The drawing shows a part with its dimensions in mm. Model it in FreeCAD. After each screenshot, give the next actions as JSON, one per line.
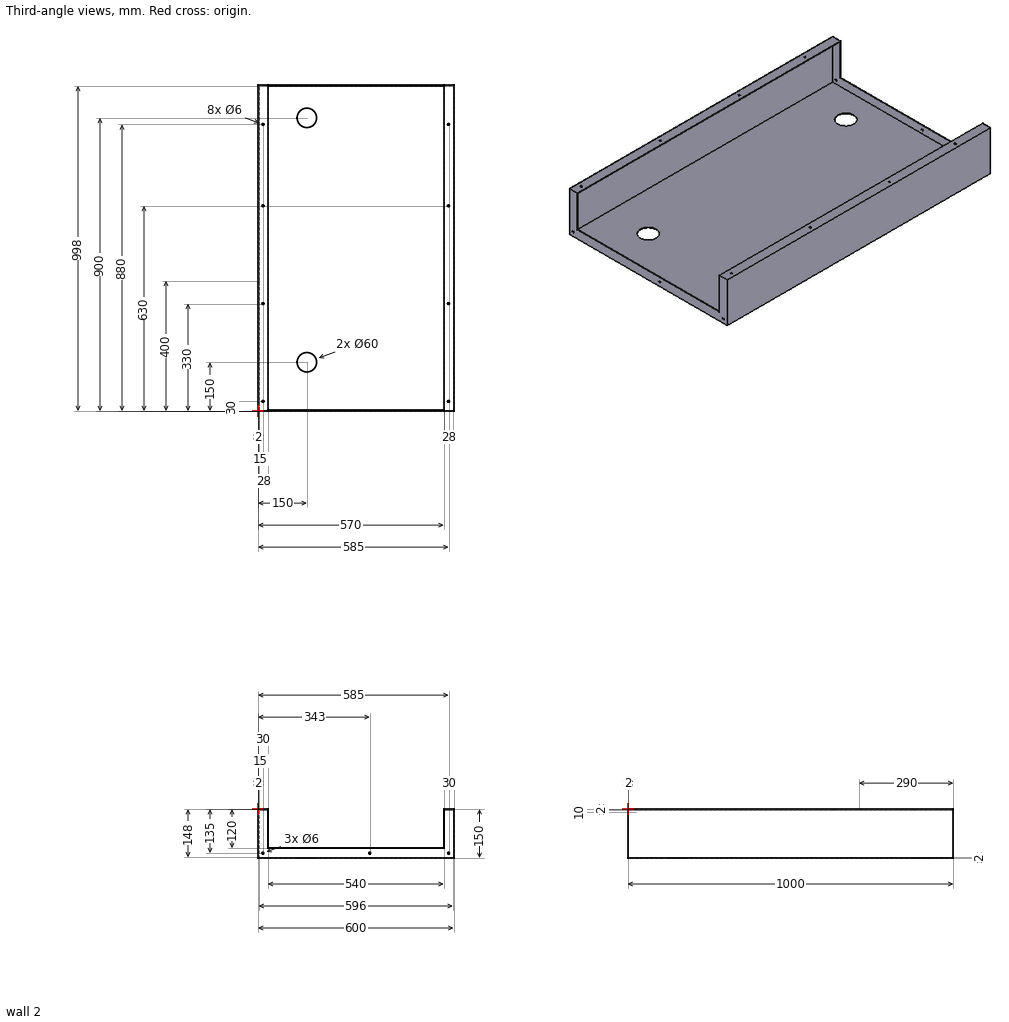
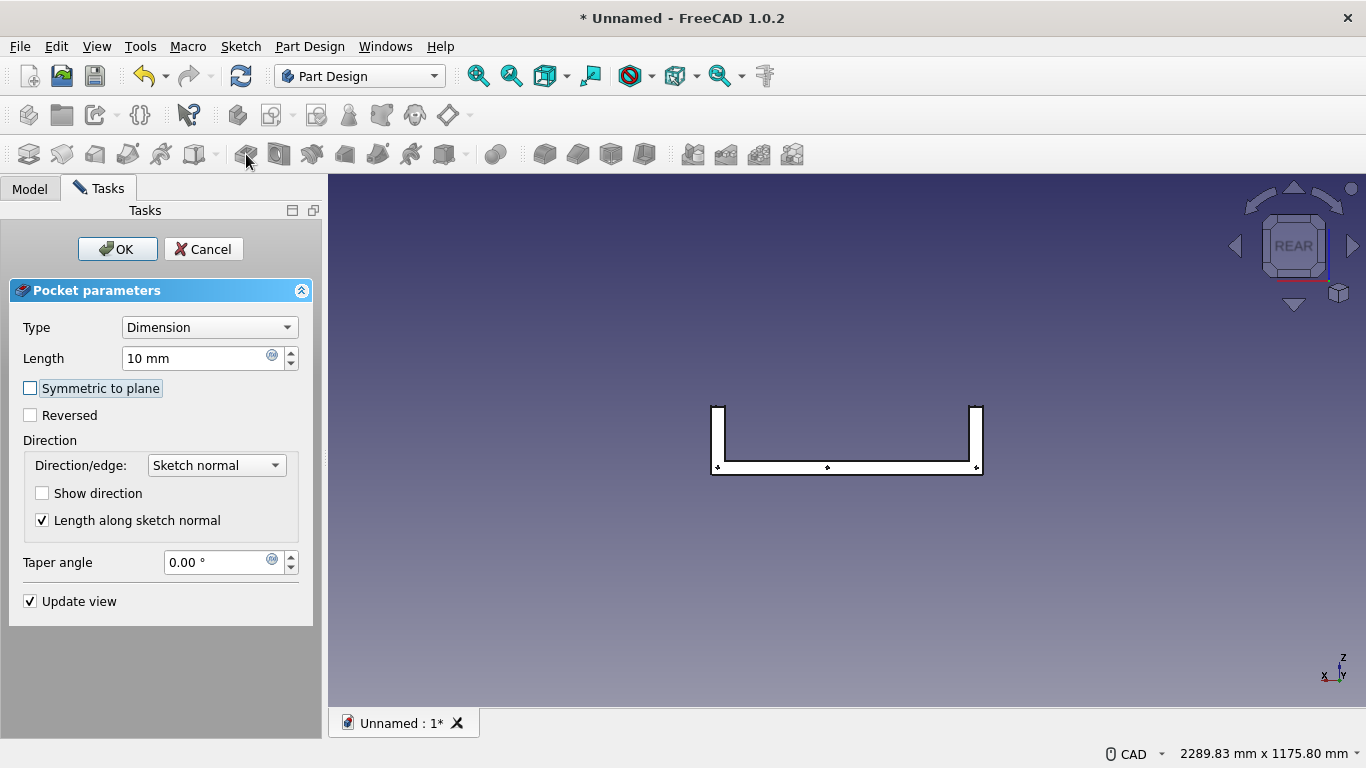
{"action": "left_click", "coordinate": [118, 249]}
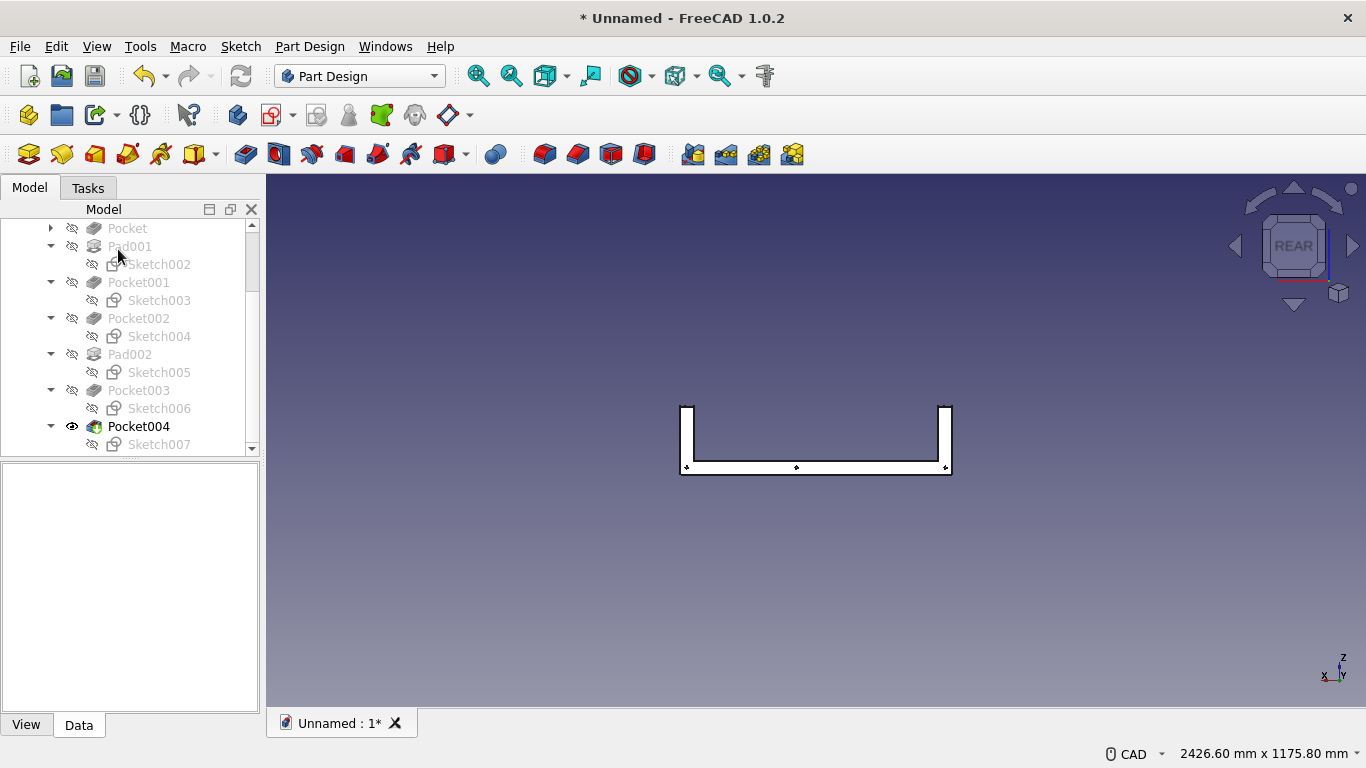
{"action": "key", "text": "0"}